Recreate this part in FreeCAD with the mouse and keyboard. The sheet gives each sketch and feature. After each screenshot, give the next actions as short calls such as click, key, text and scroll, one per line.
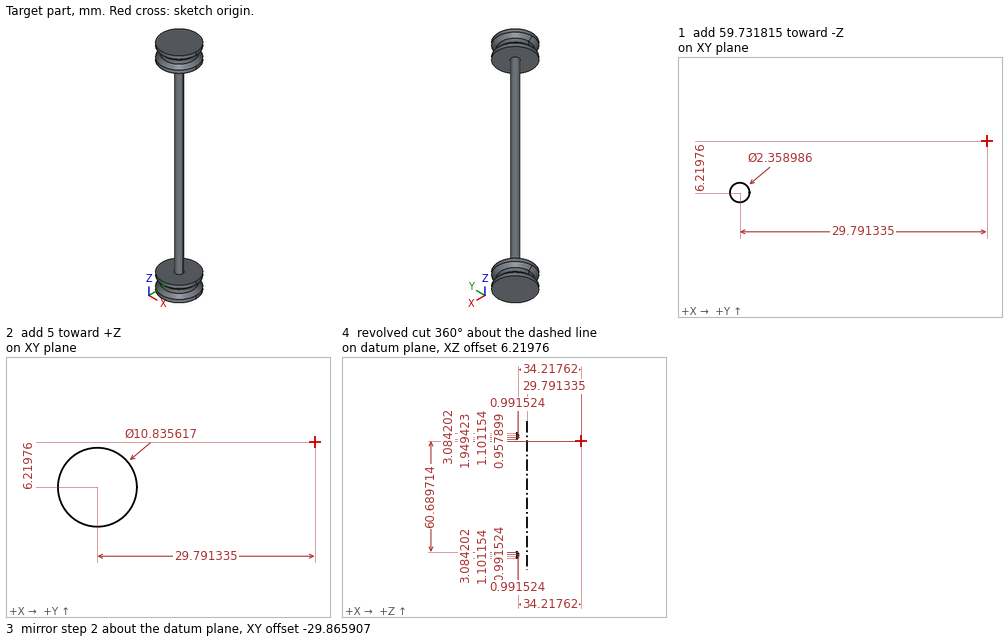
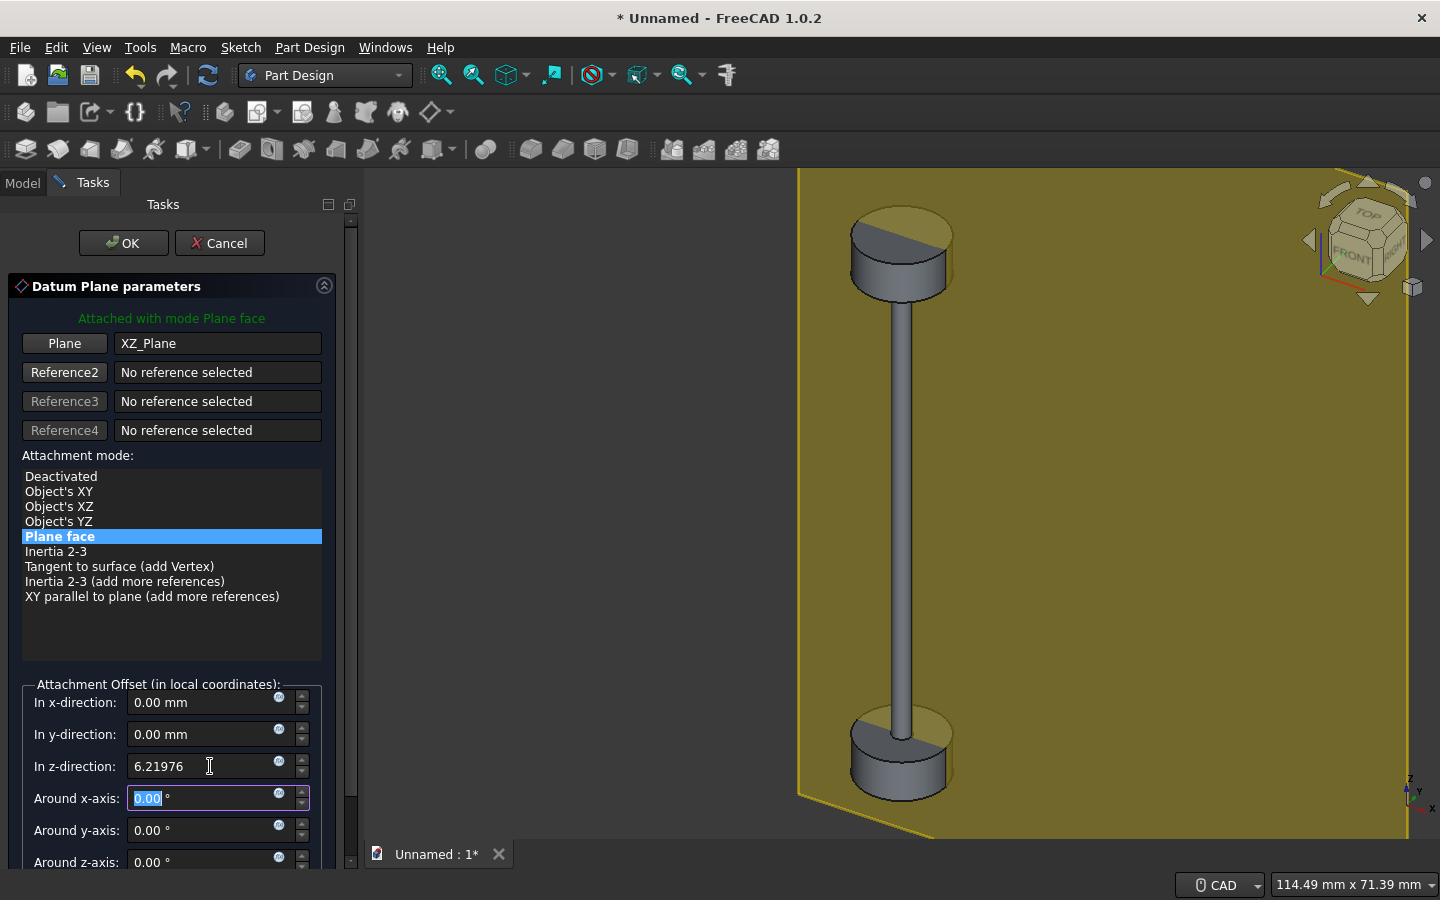
click(124, 243)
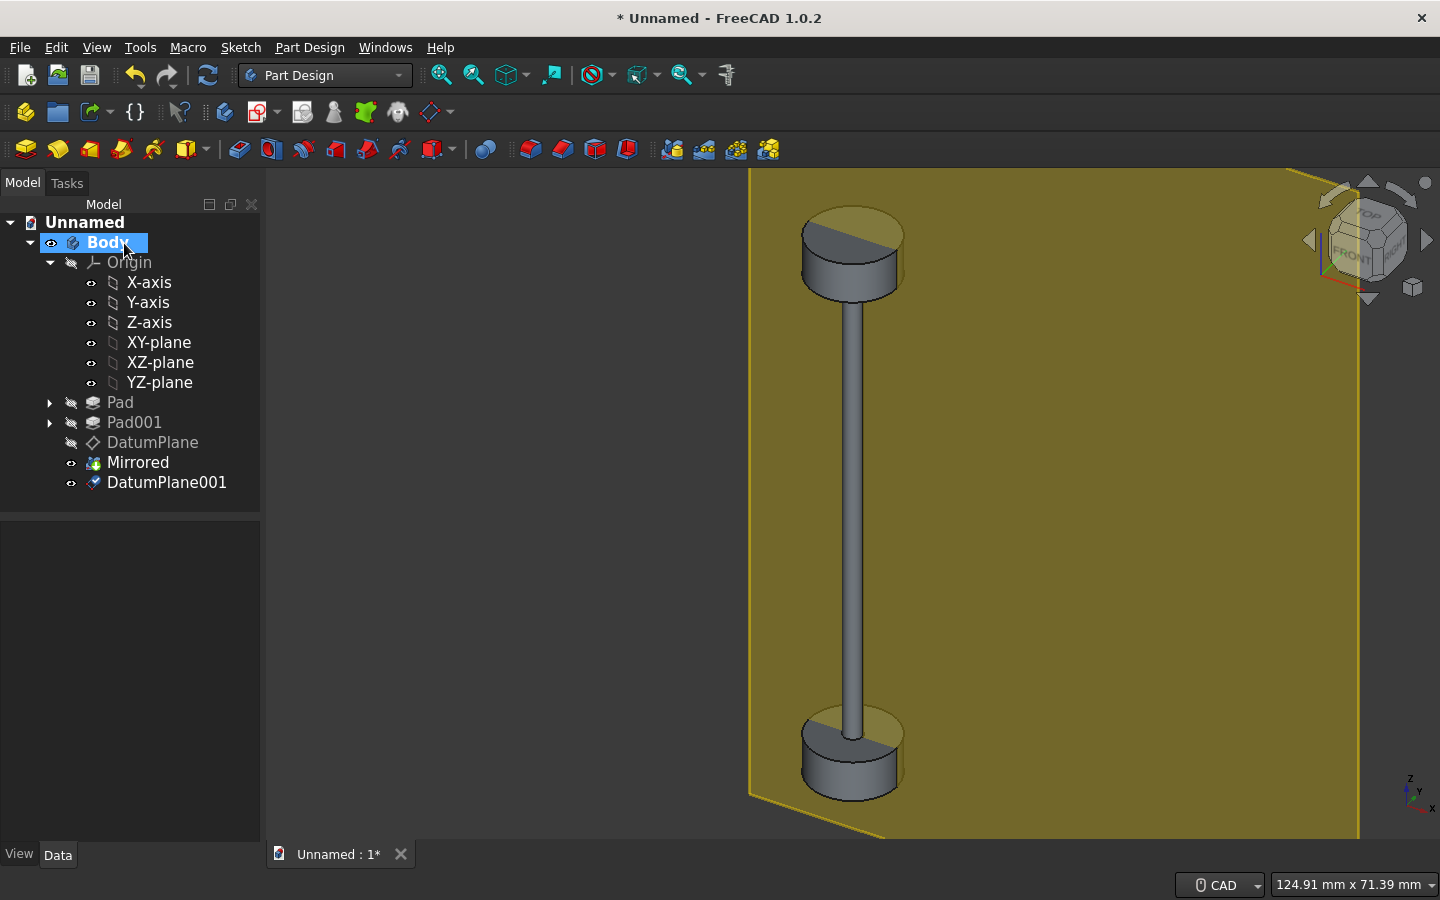
click(116, 483)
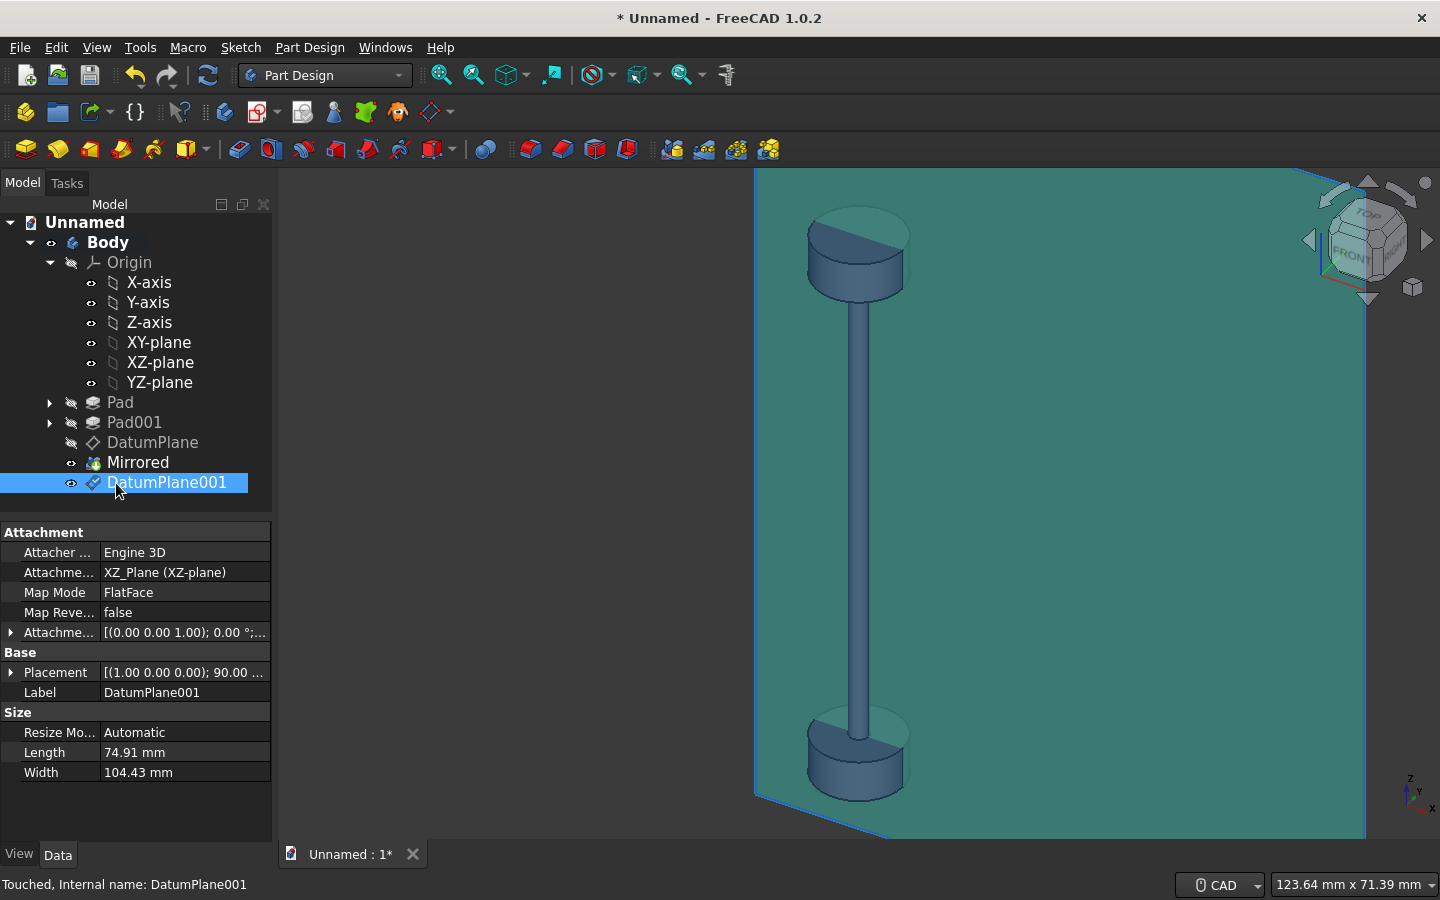
click(258, 112)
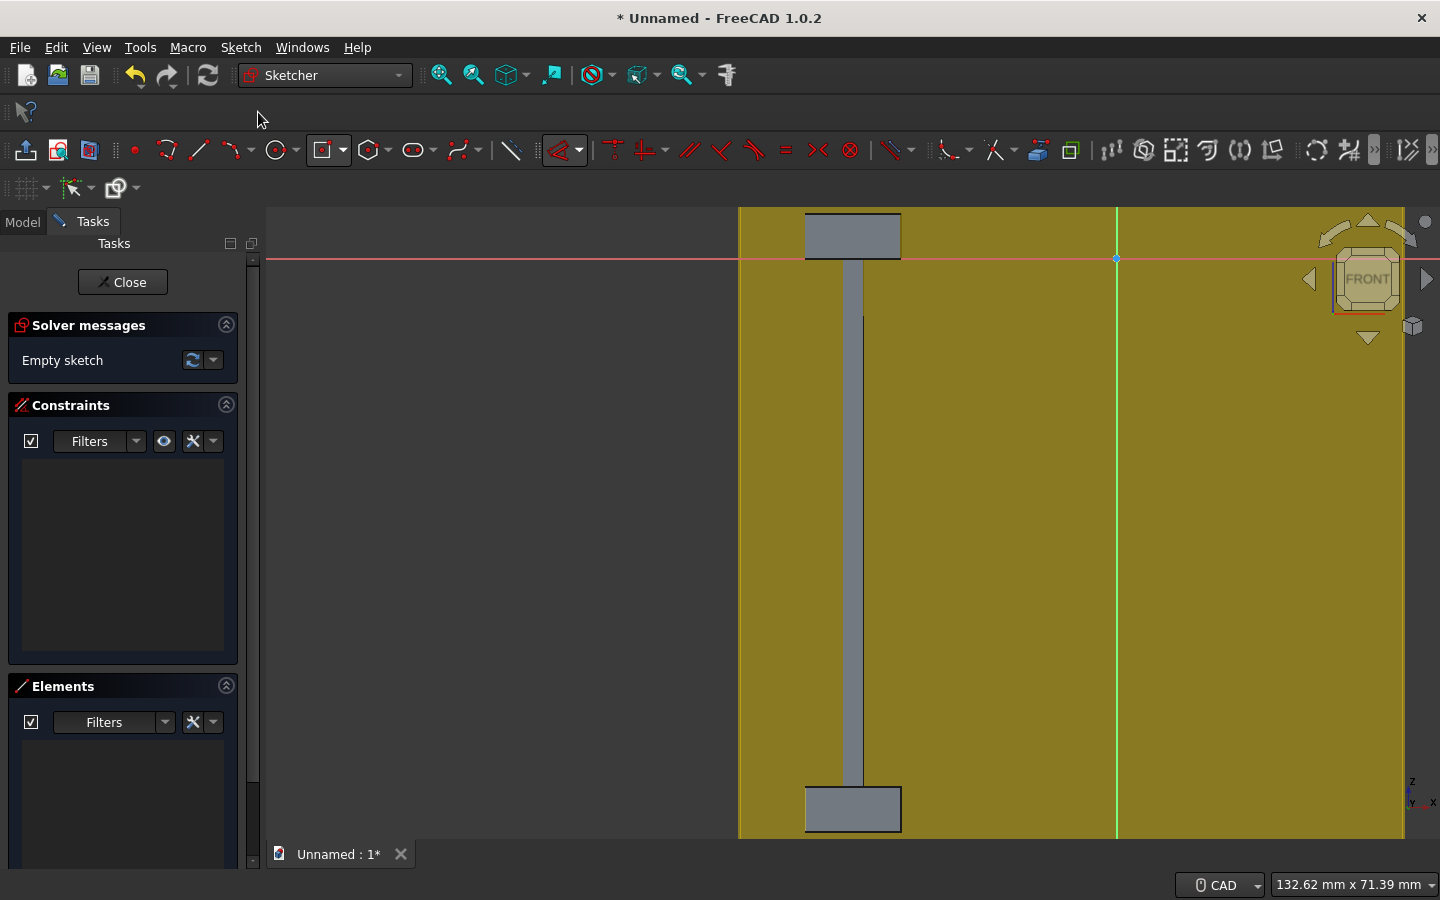
key(q)
key(s)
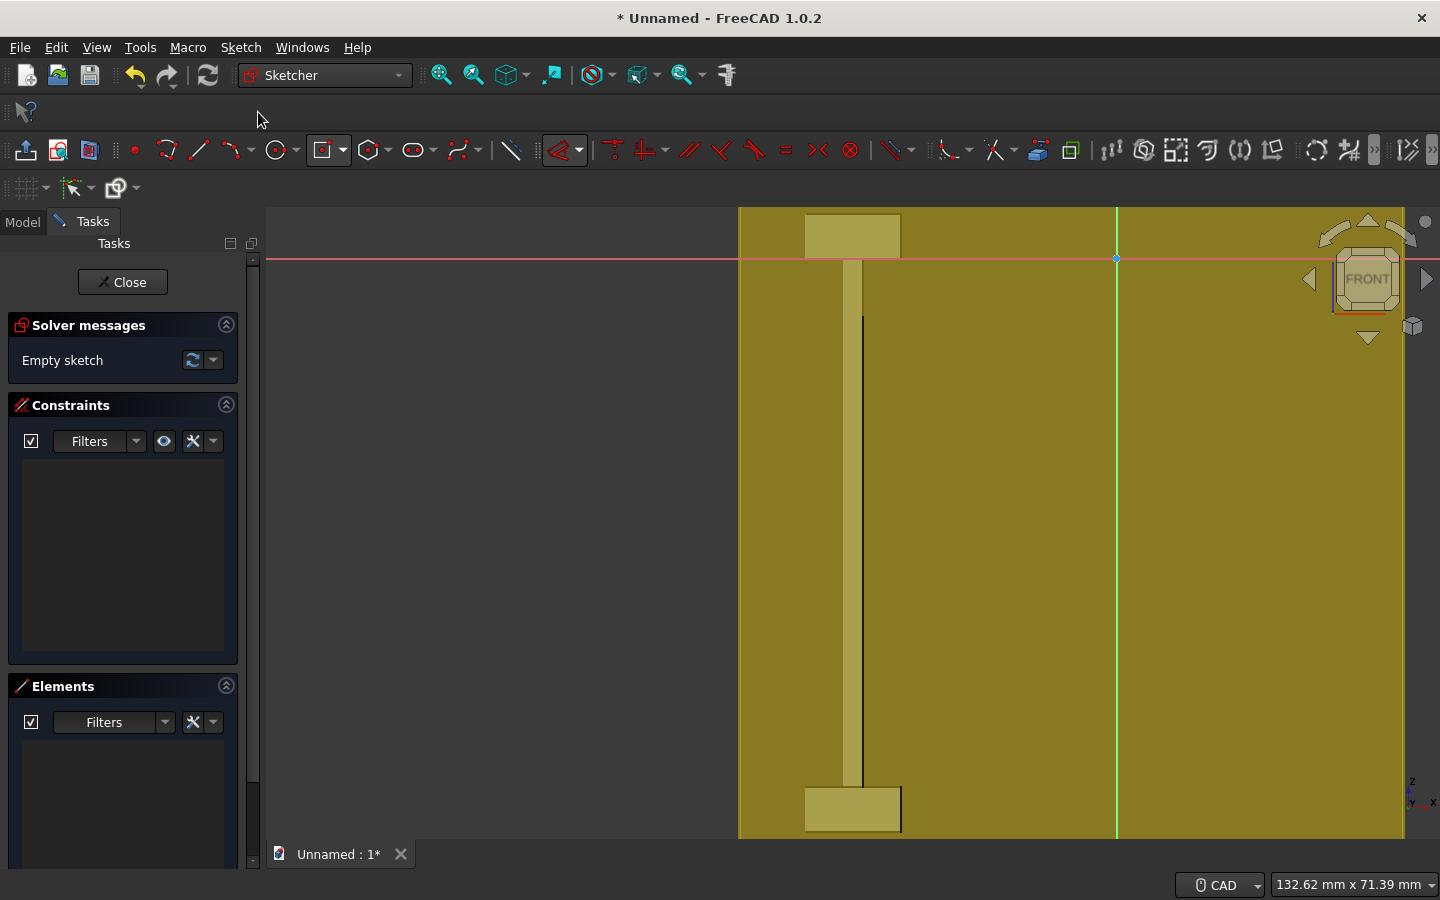
scroll(570, 523, down, 3)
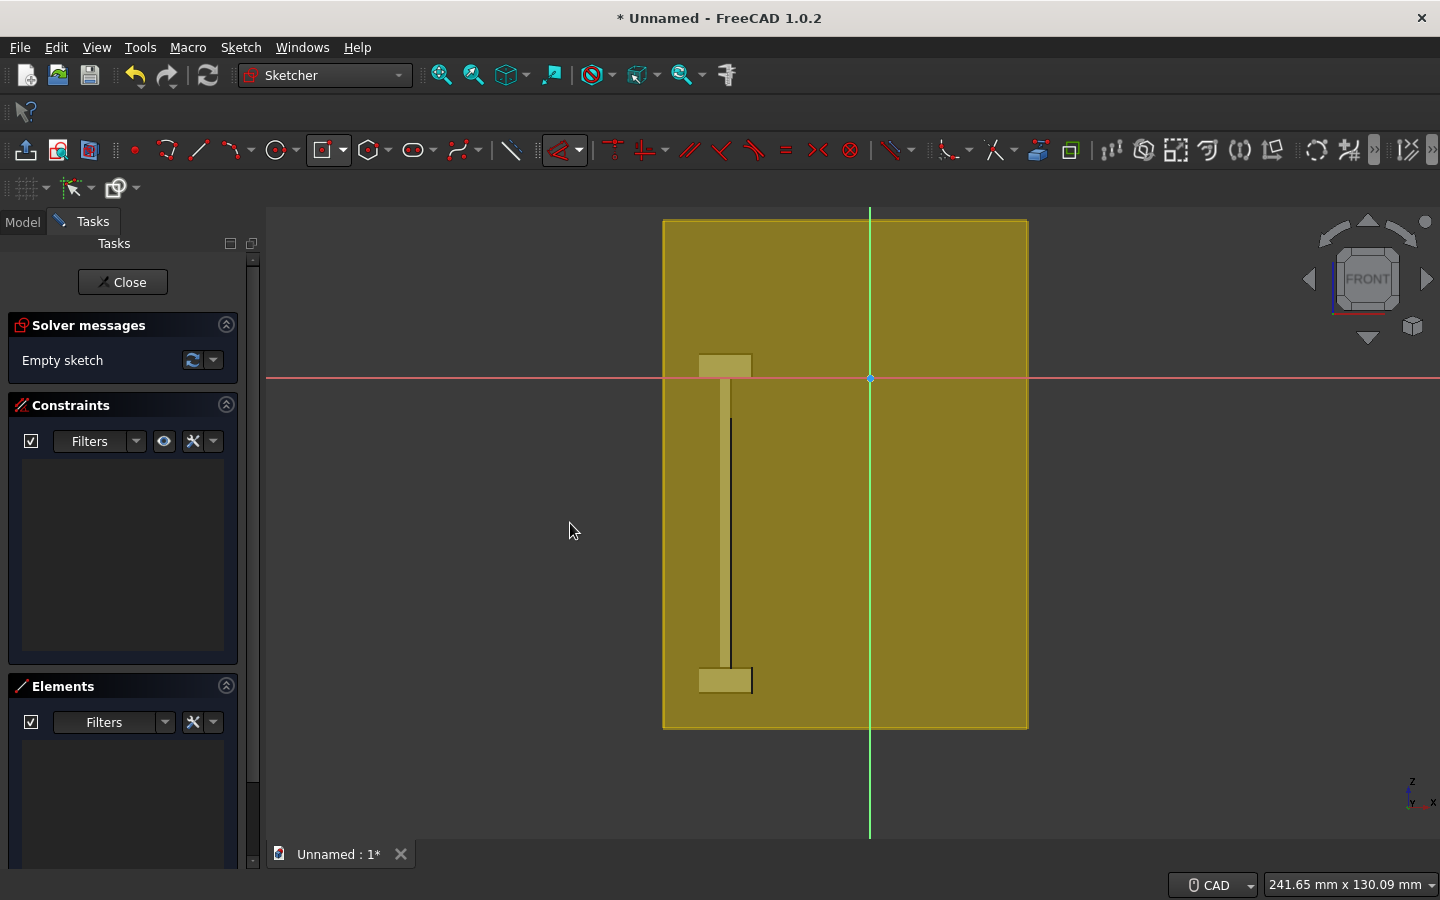
key(g)
key(m)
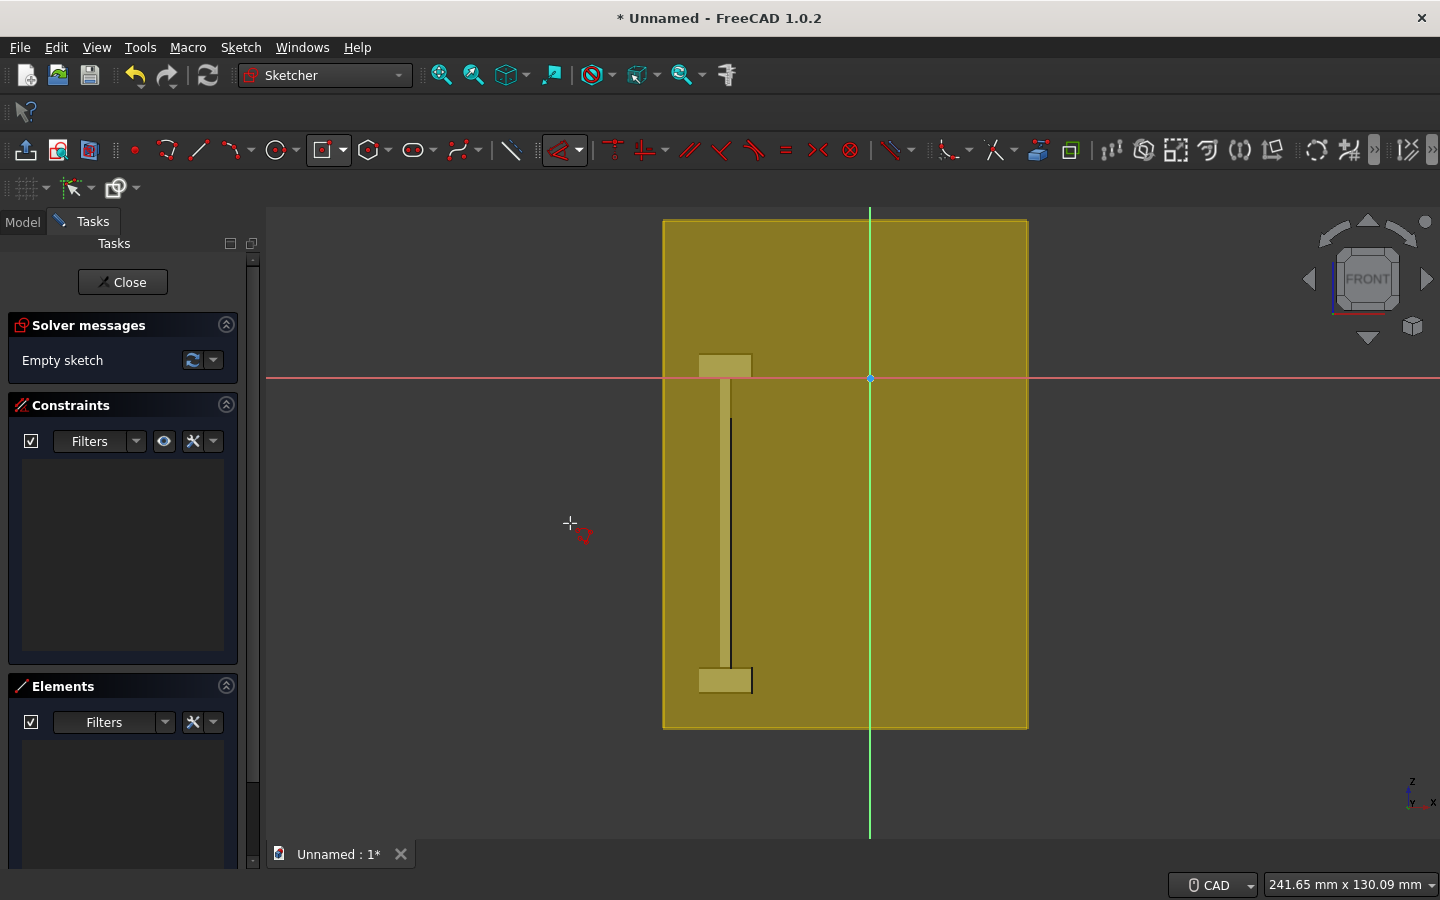
scroll(704, 369, up, 3)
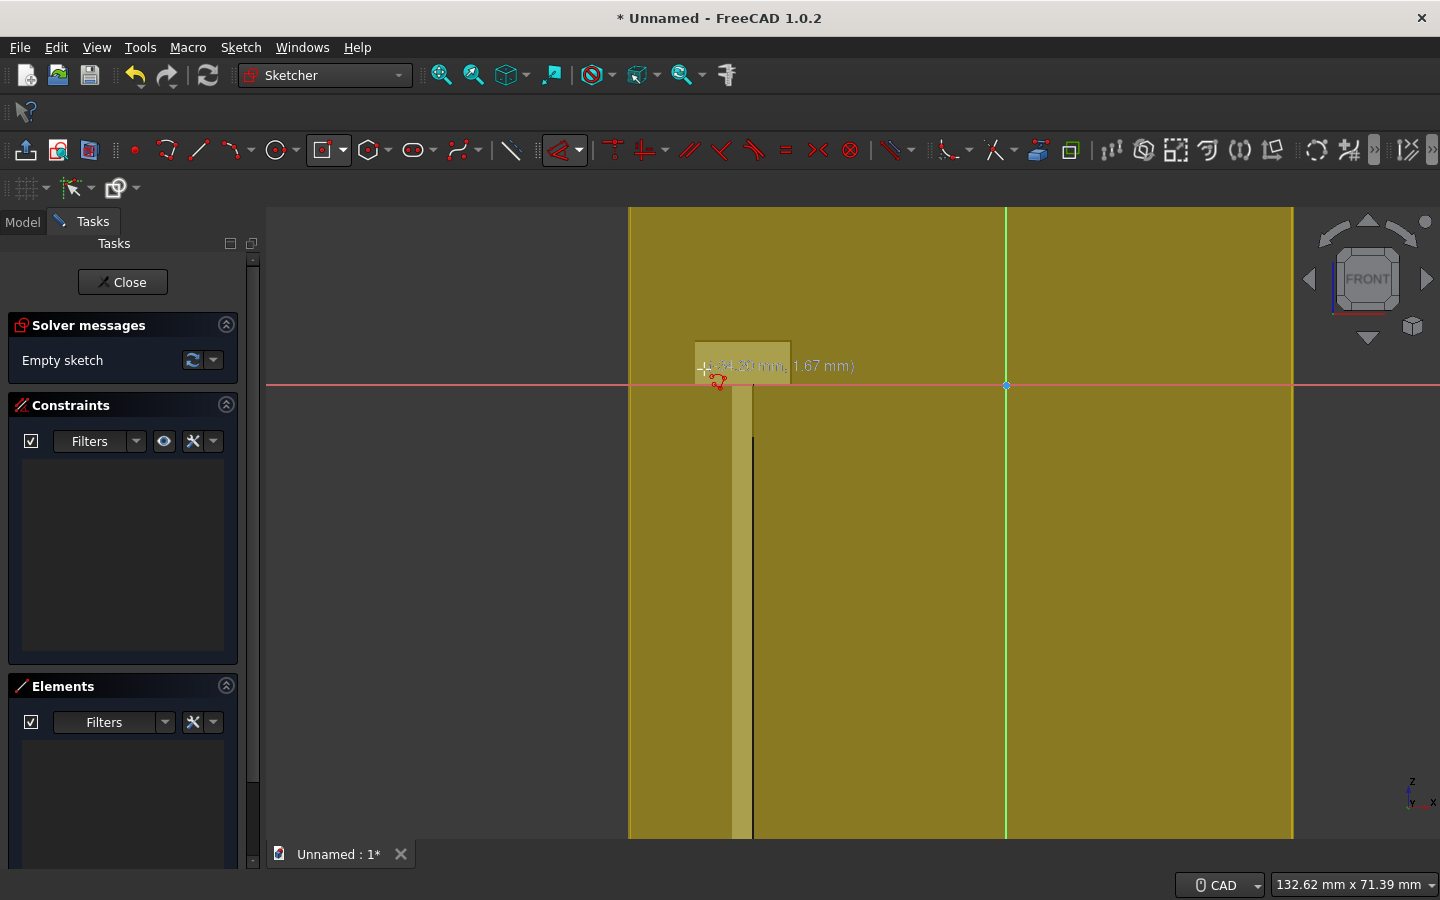
click(704, 368)